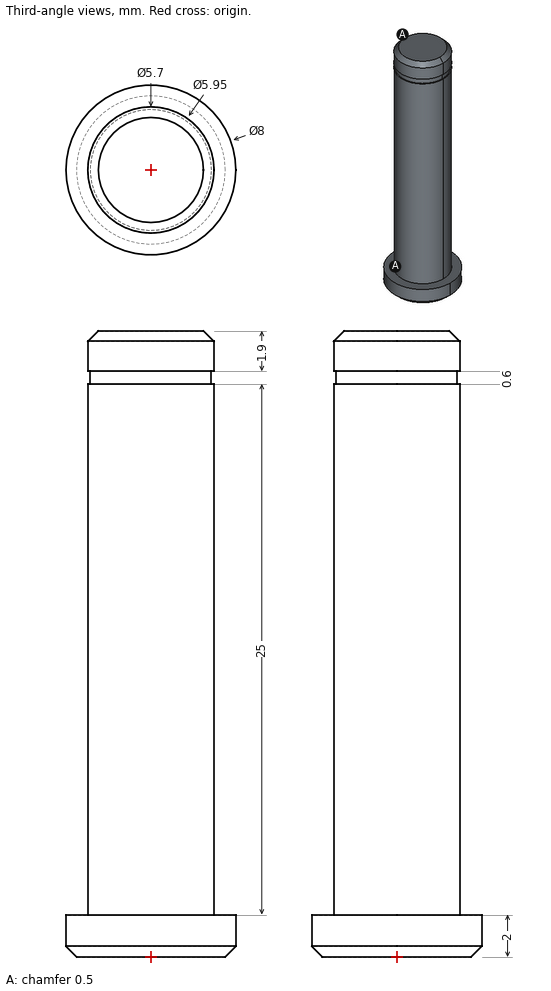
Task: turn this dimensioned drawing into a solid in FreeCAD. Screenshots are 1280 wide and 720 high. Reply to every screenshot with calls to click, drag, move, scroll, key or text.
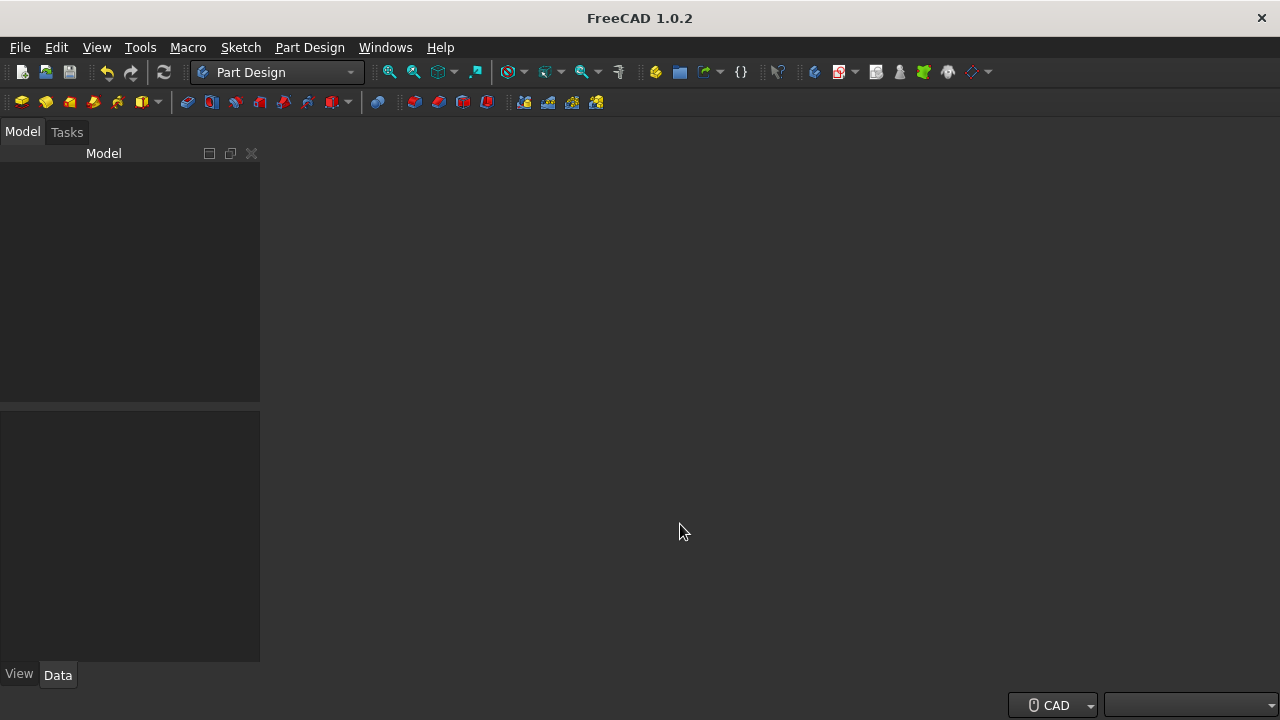
key(ctrl+n)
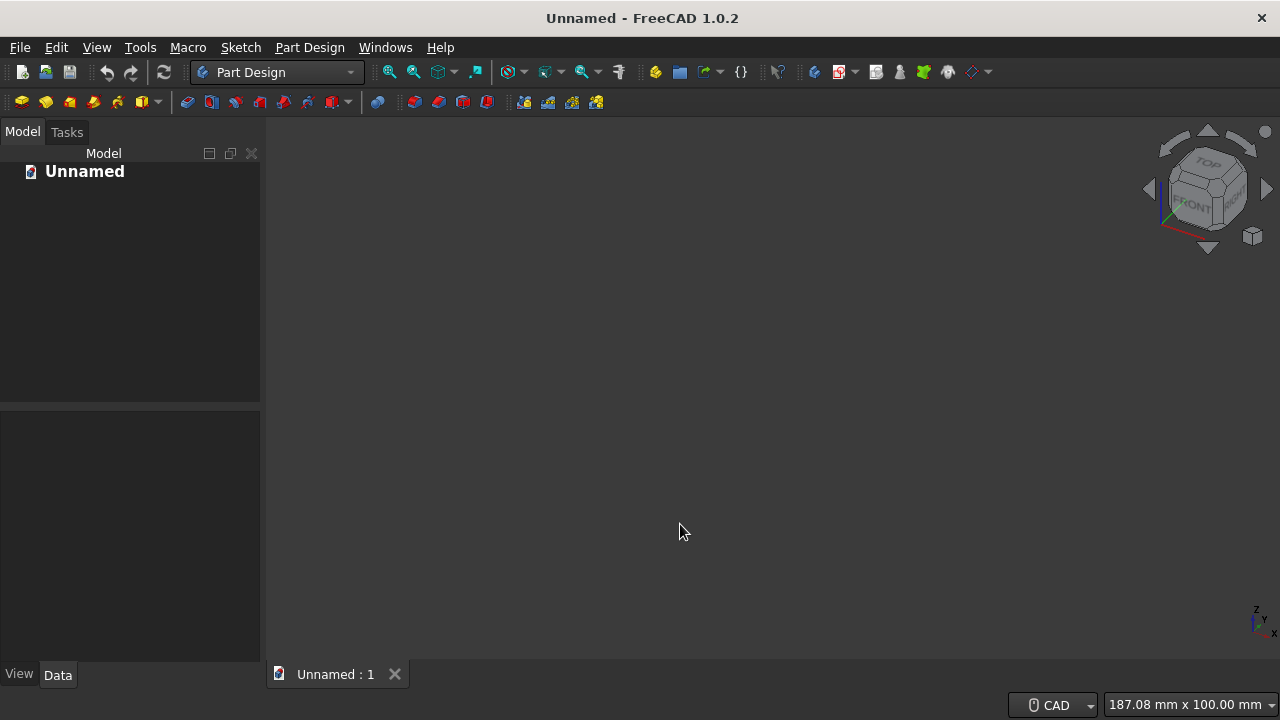
click(840, 72)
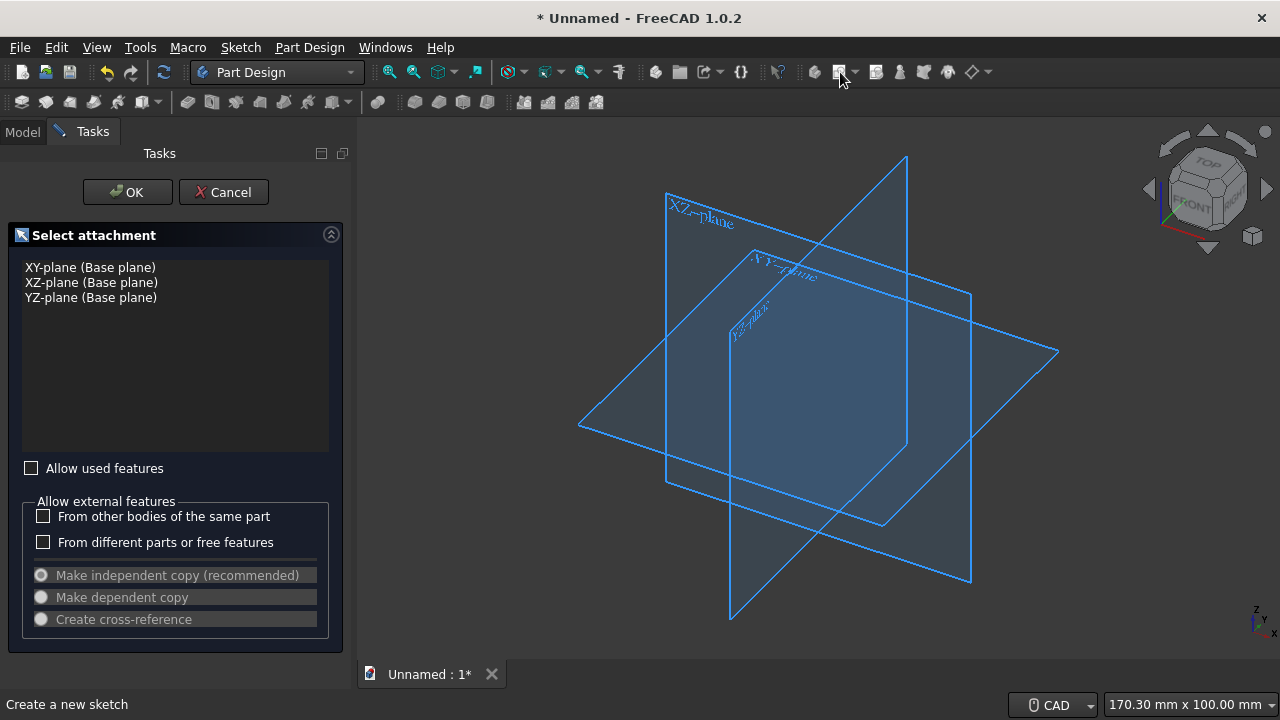
click(82, 268)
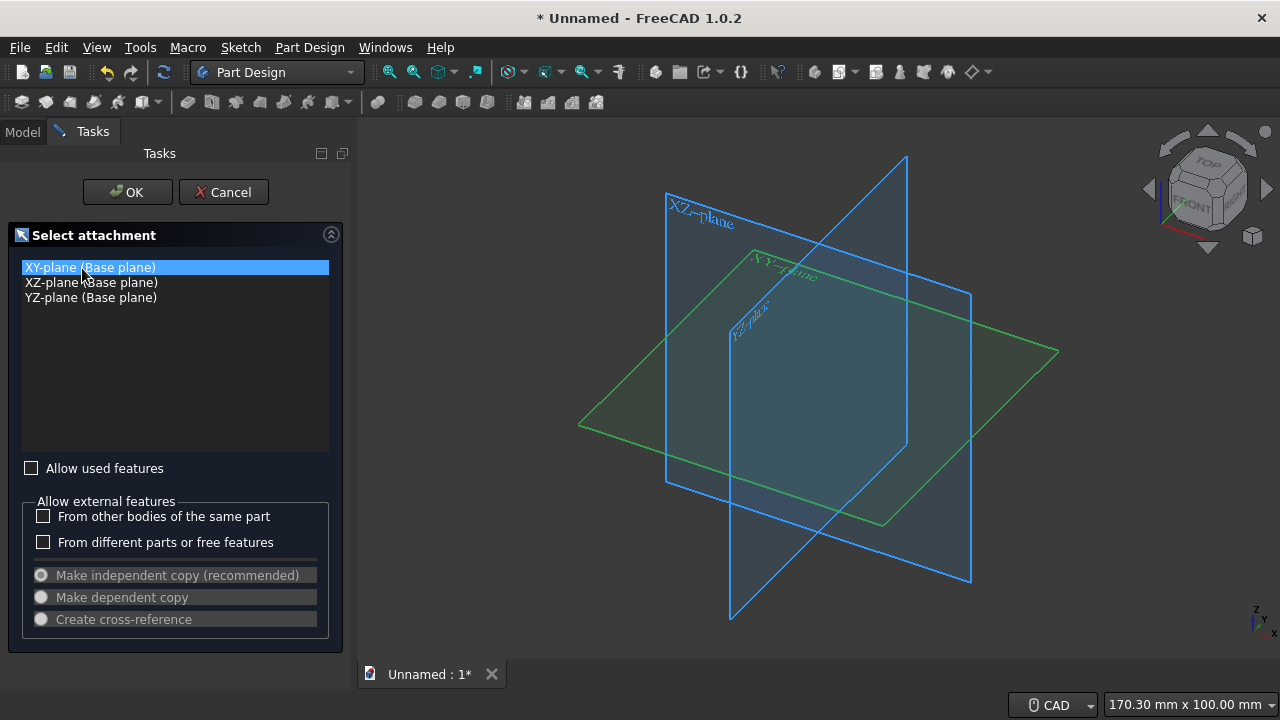
click(128, 192)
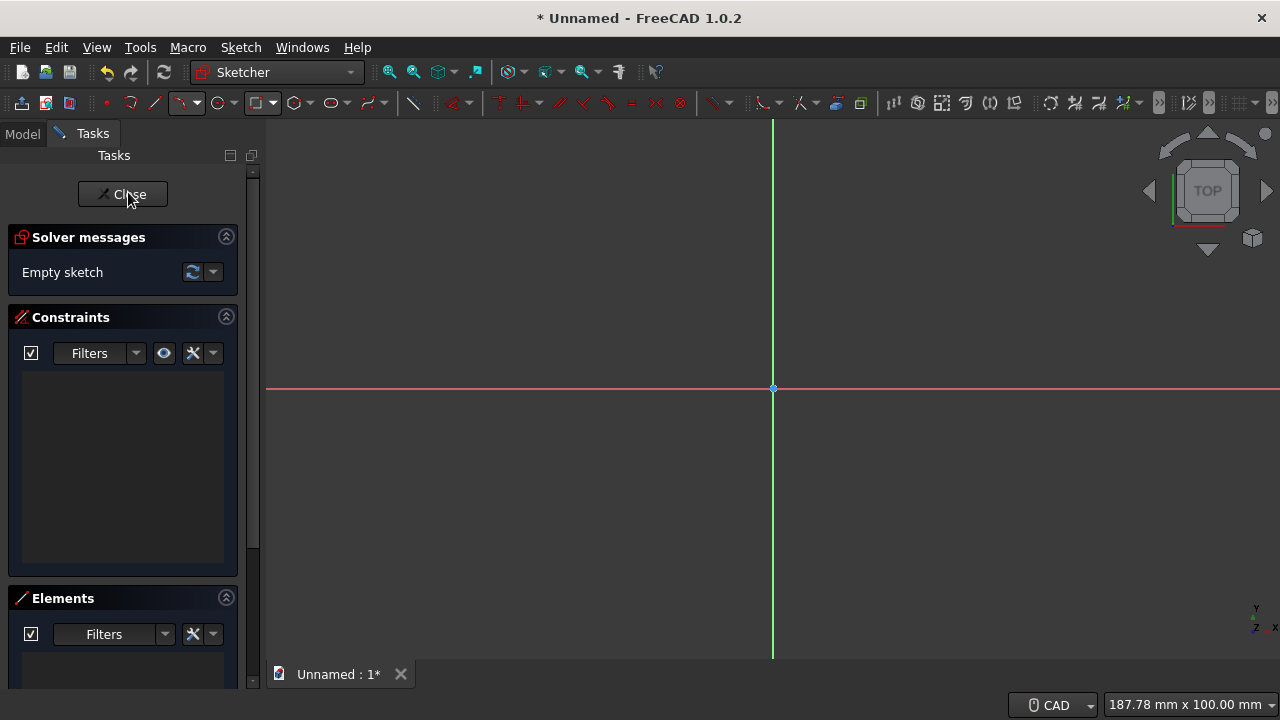
scroll(784, 389, up, 10)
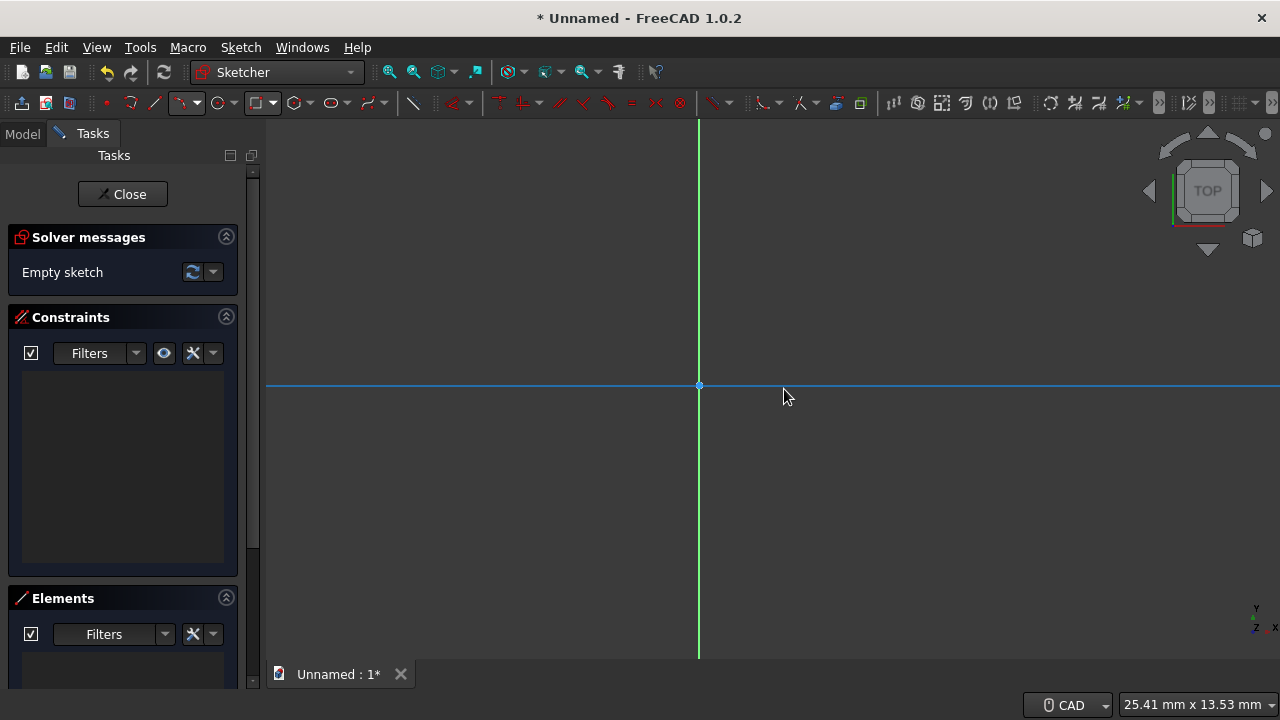
key(g)
key(c)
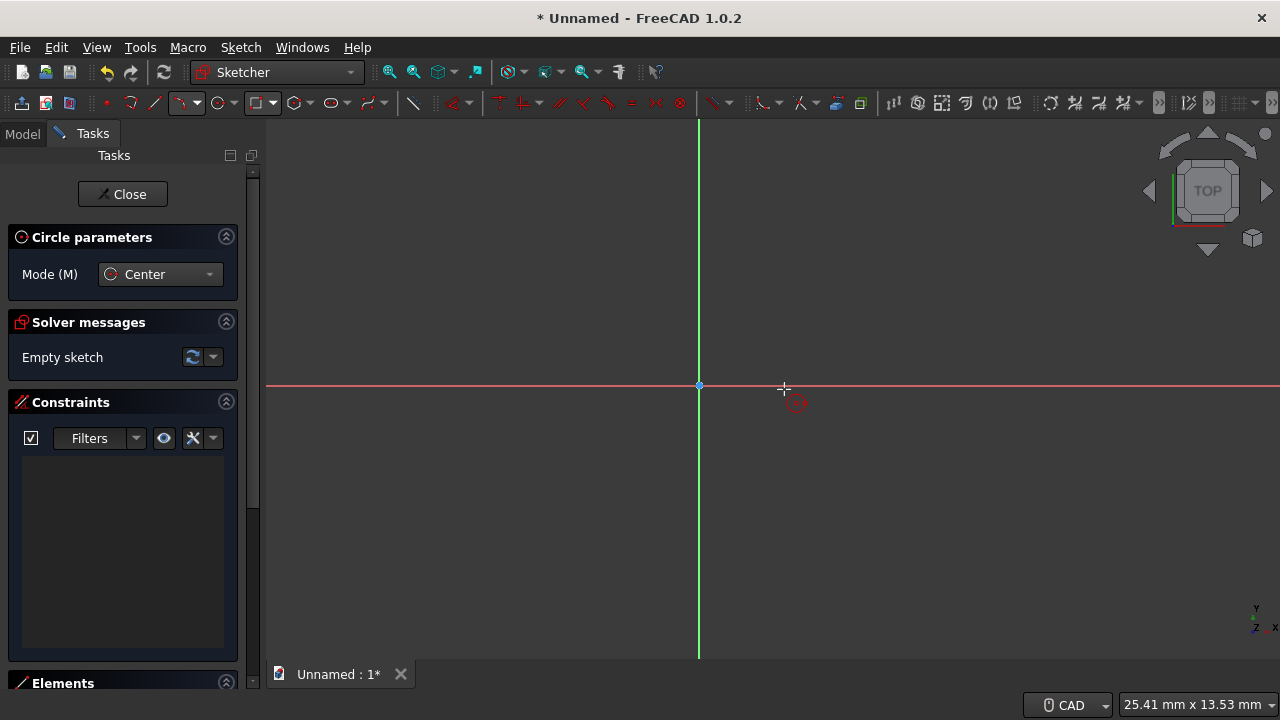
click(699, 386)
move(812, 273)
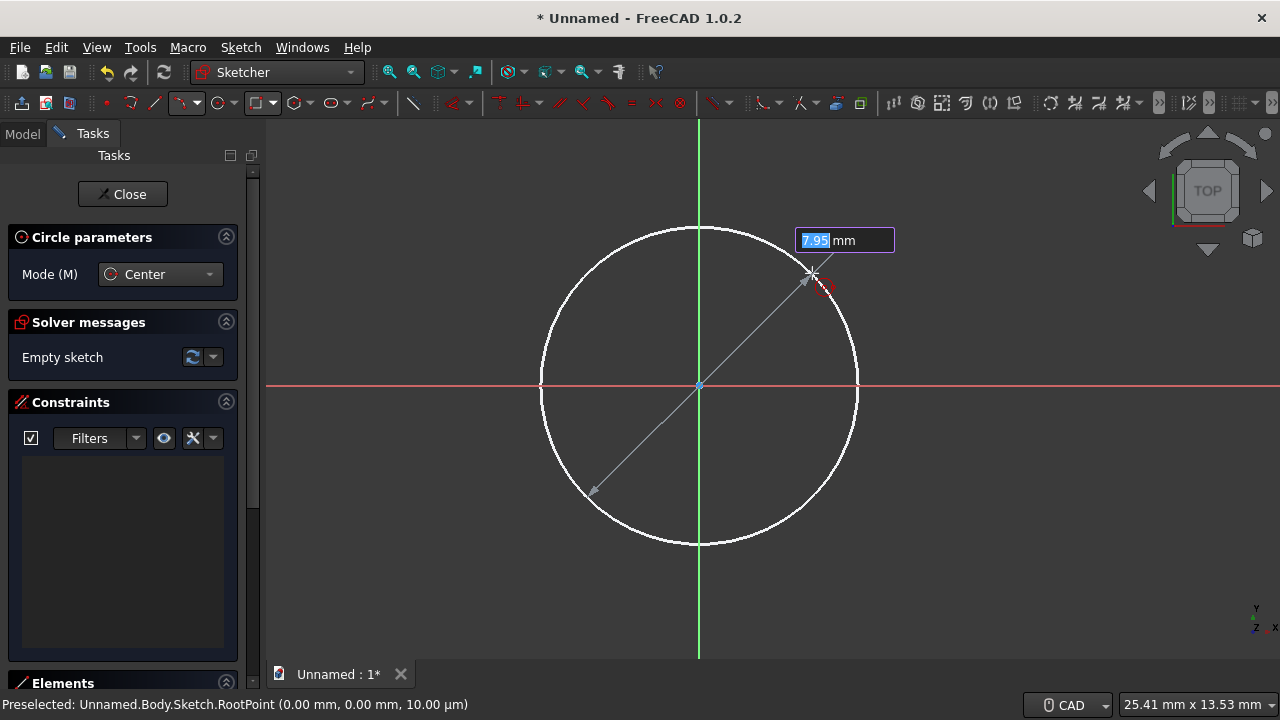
text(8)
key(Return)
key(Escape)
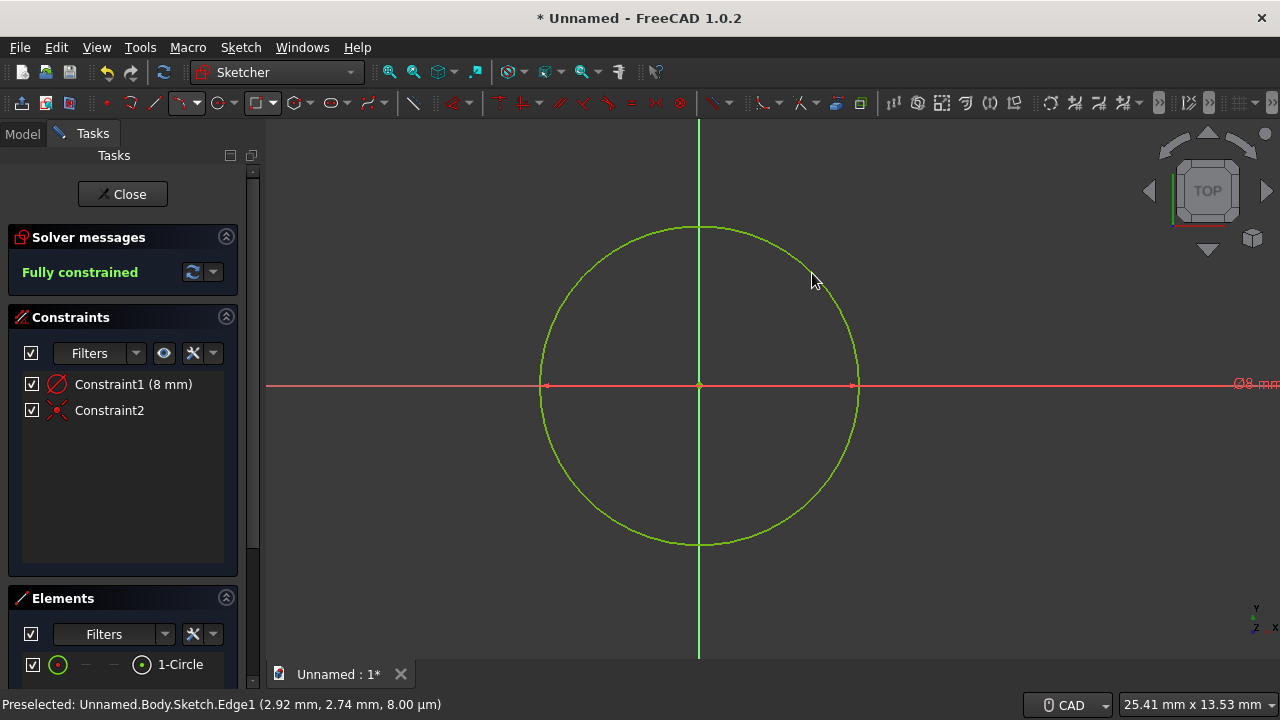
click(123, 194)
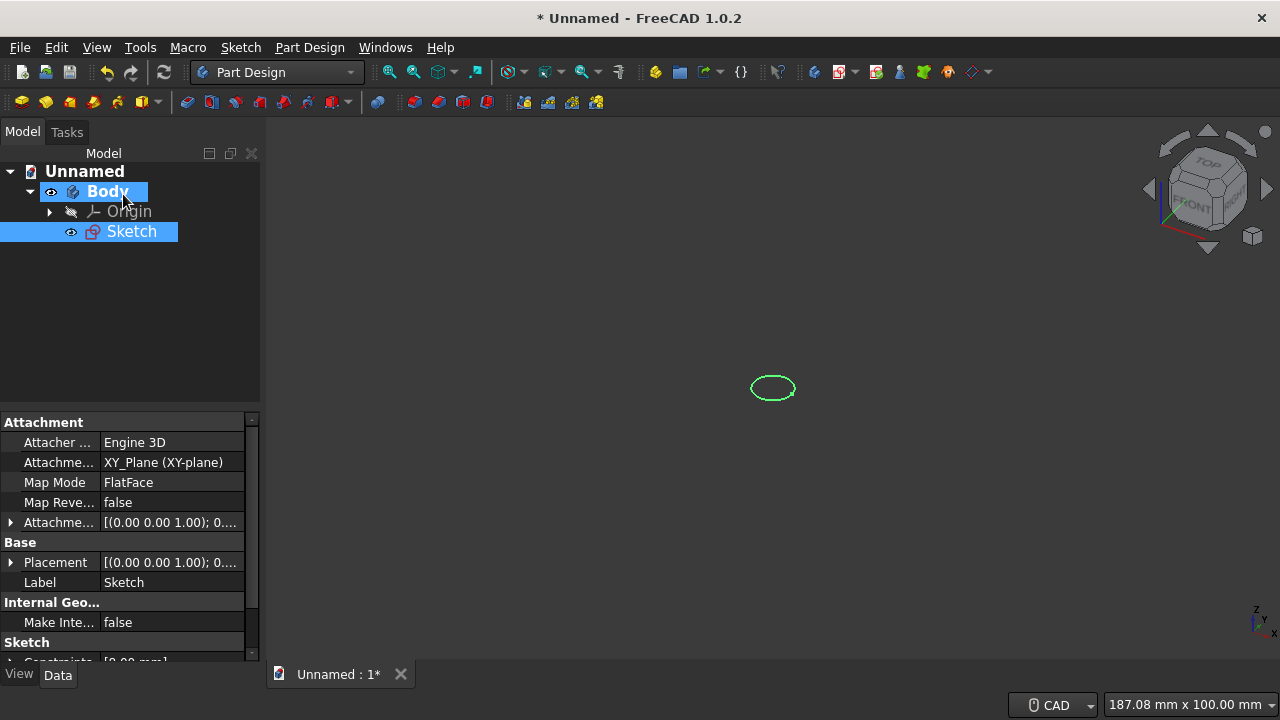
click(22, 102)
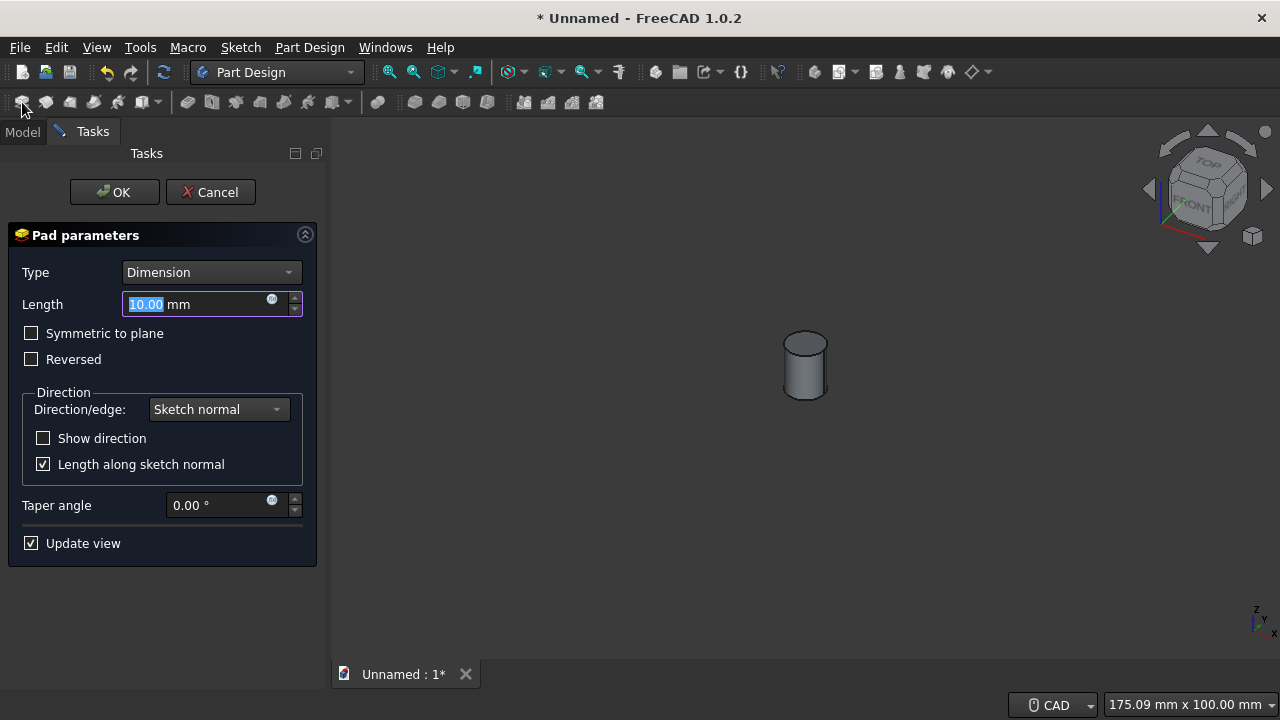
text(2)
key(Tab)